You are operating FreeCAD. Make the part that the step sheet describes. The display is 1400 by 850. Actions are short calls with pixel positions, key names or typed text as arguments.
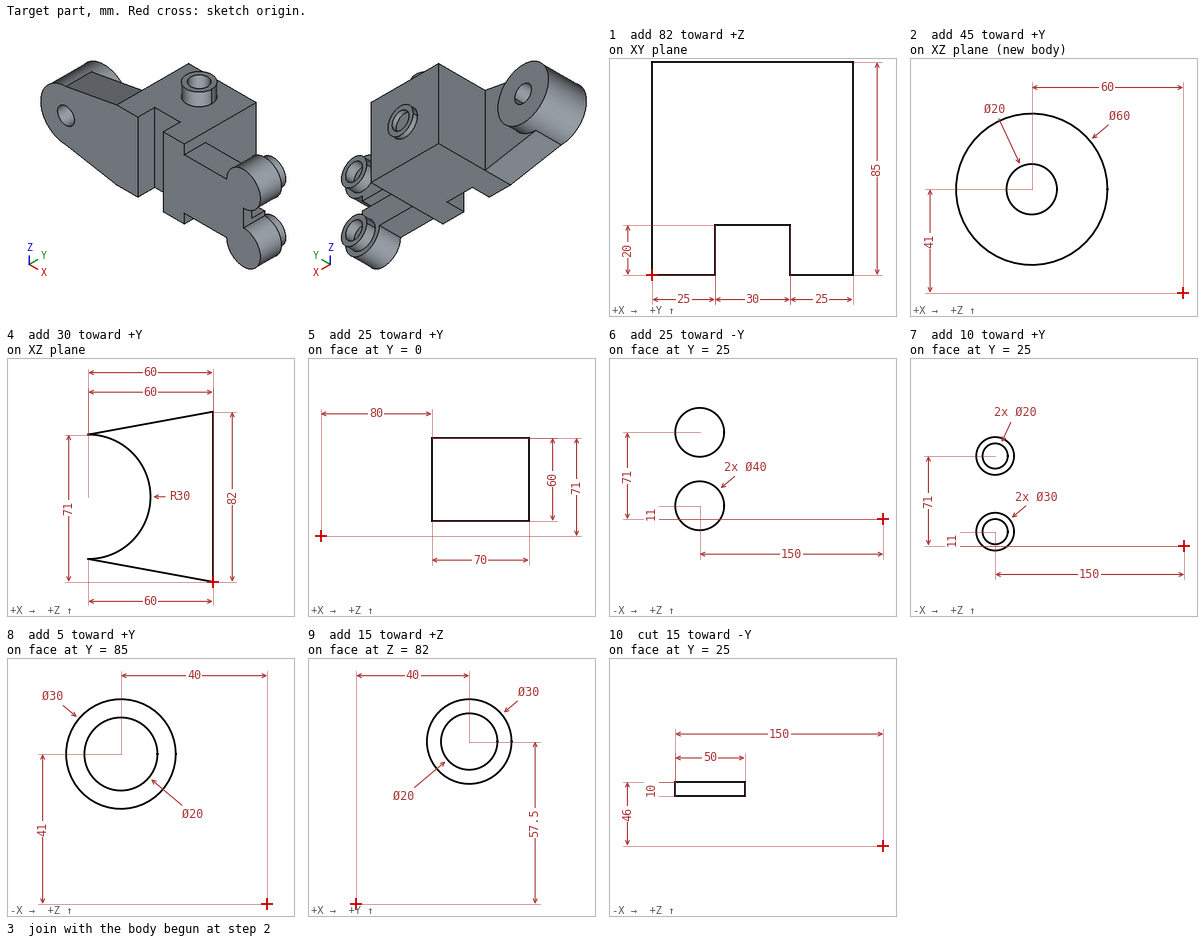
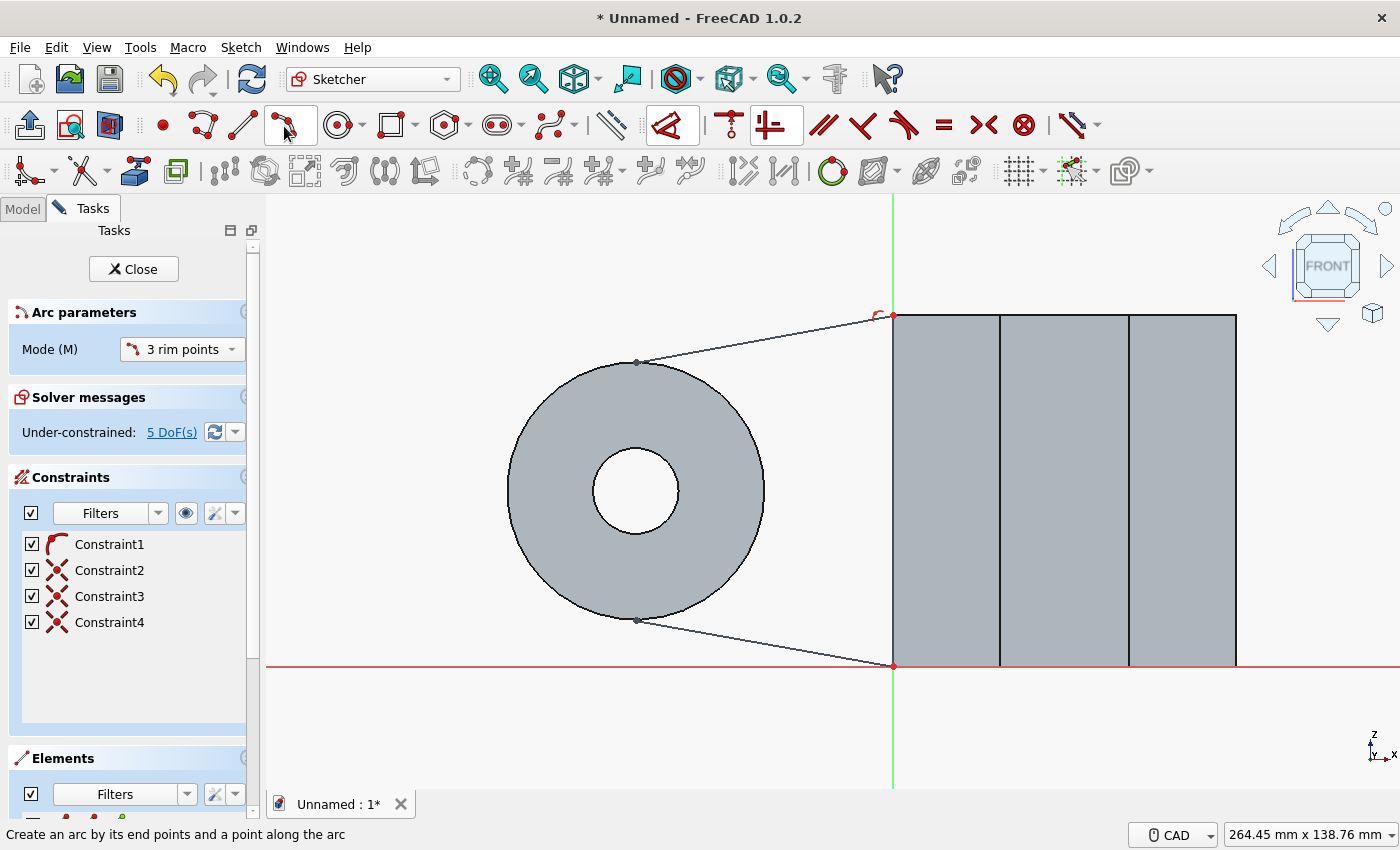
click(636, 621)
click(636, 363)
click(764, 491)
key(Escape)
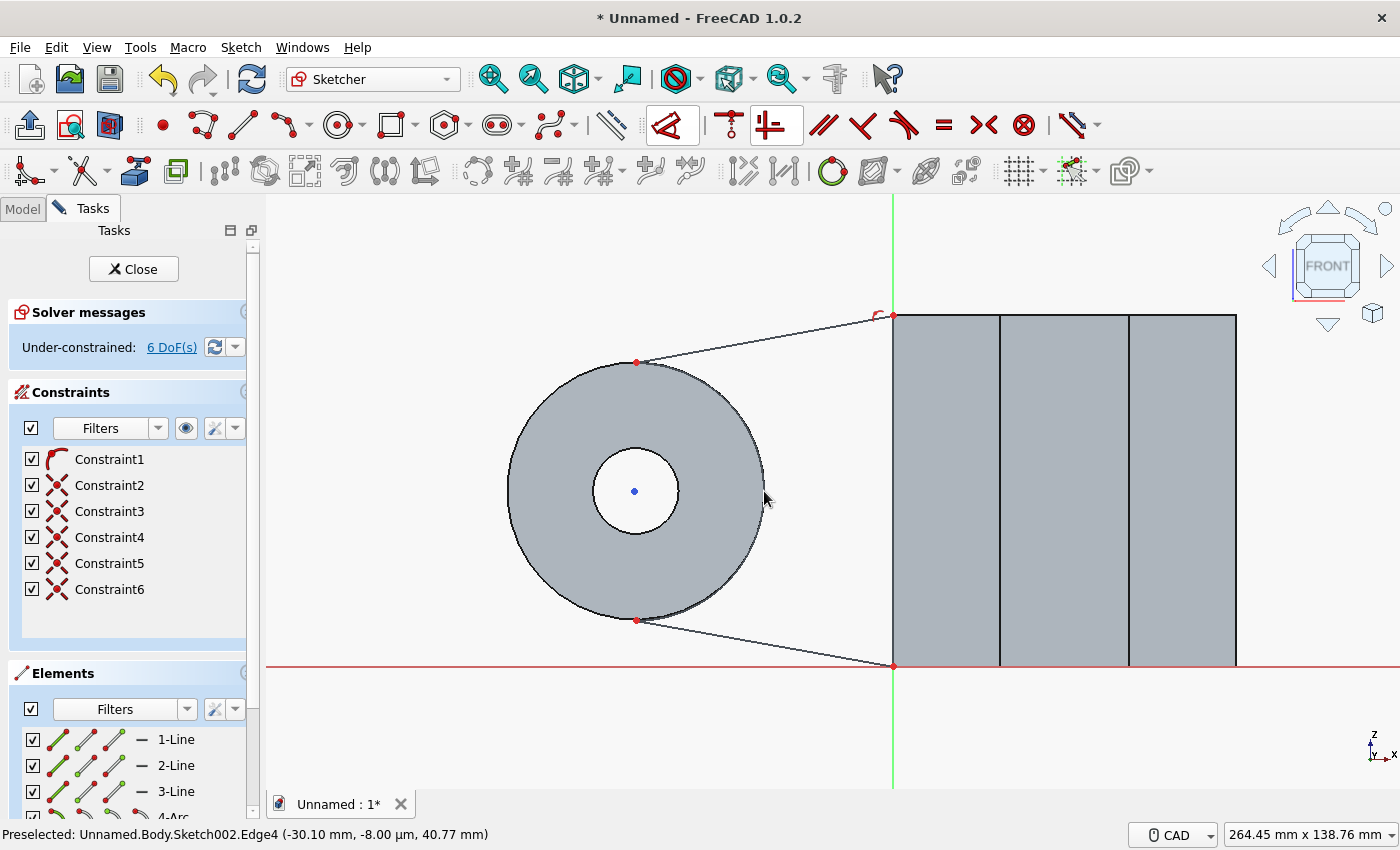
click(740, 568)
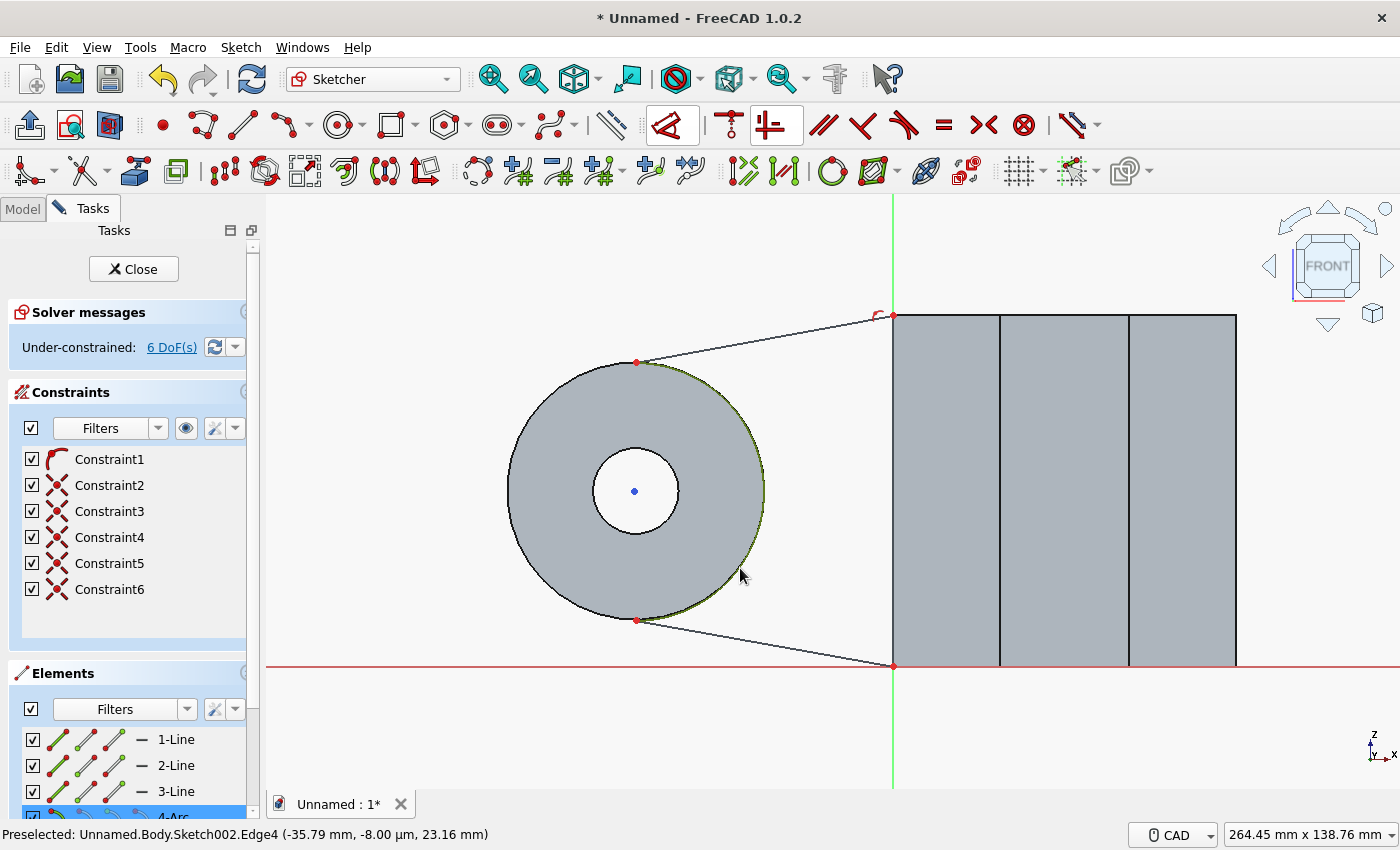
key(k)
key(r)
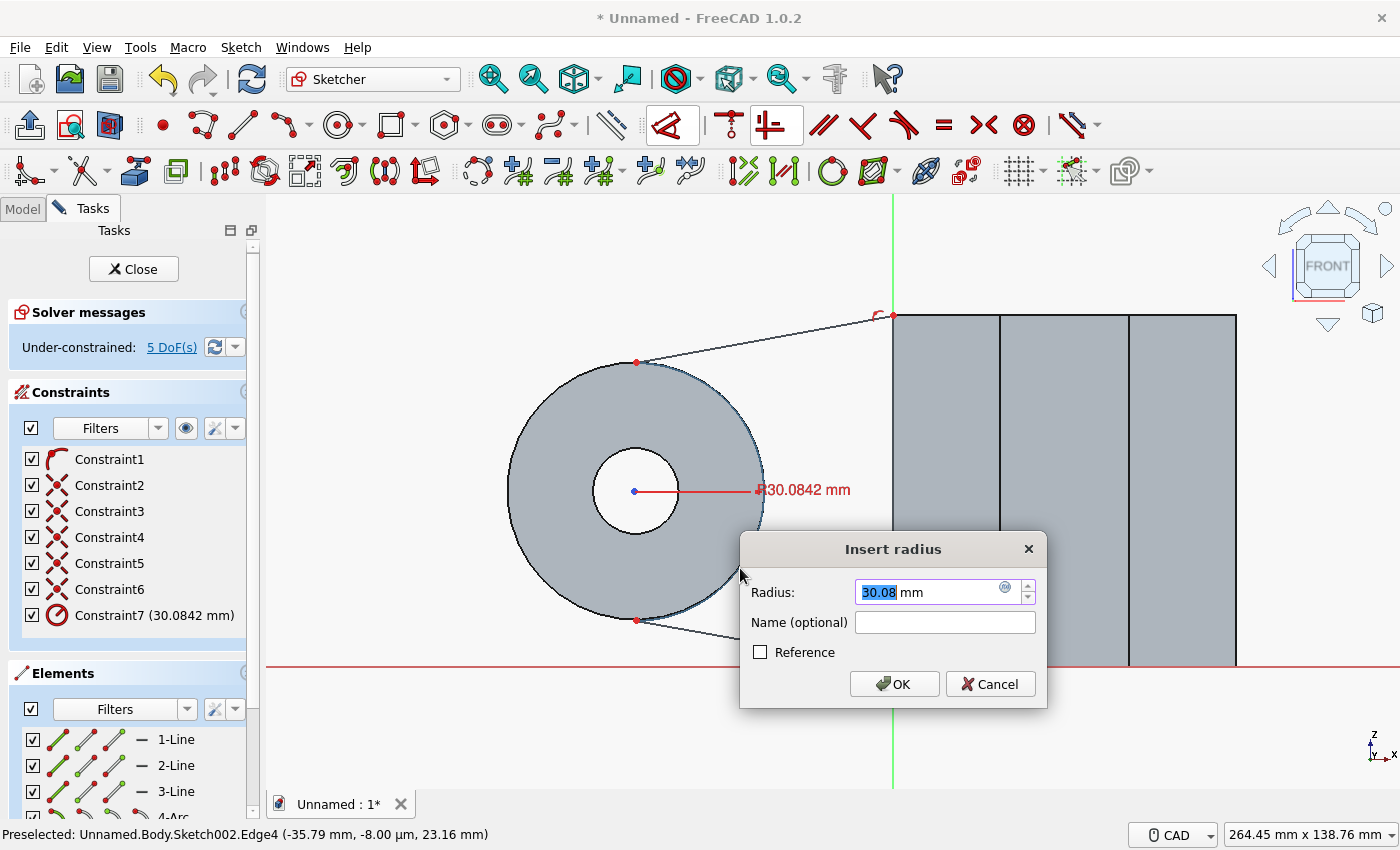
text(30)
key(Return)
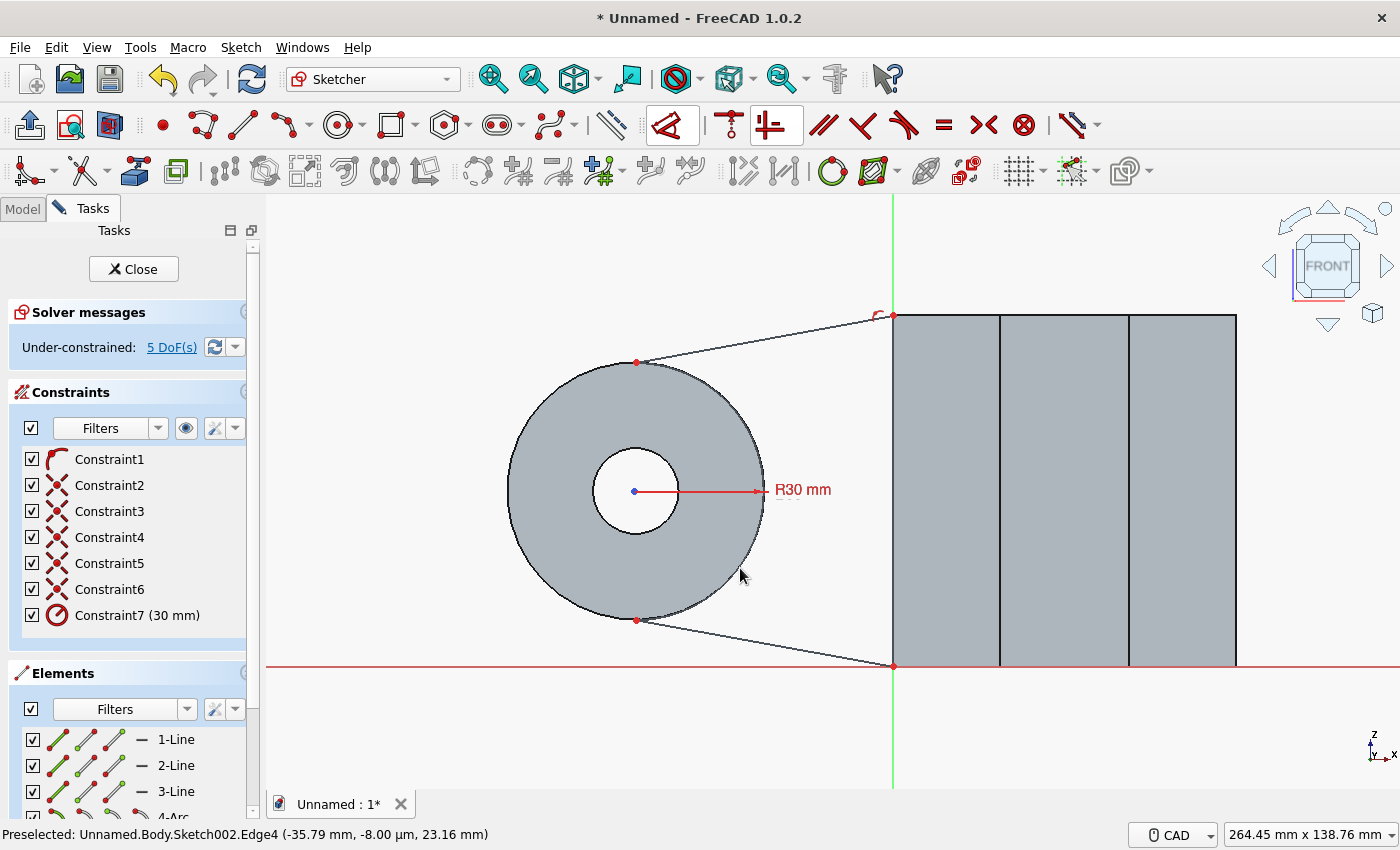
click(893, 421)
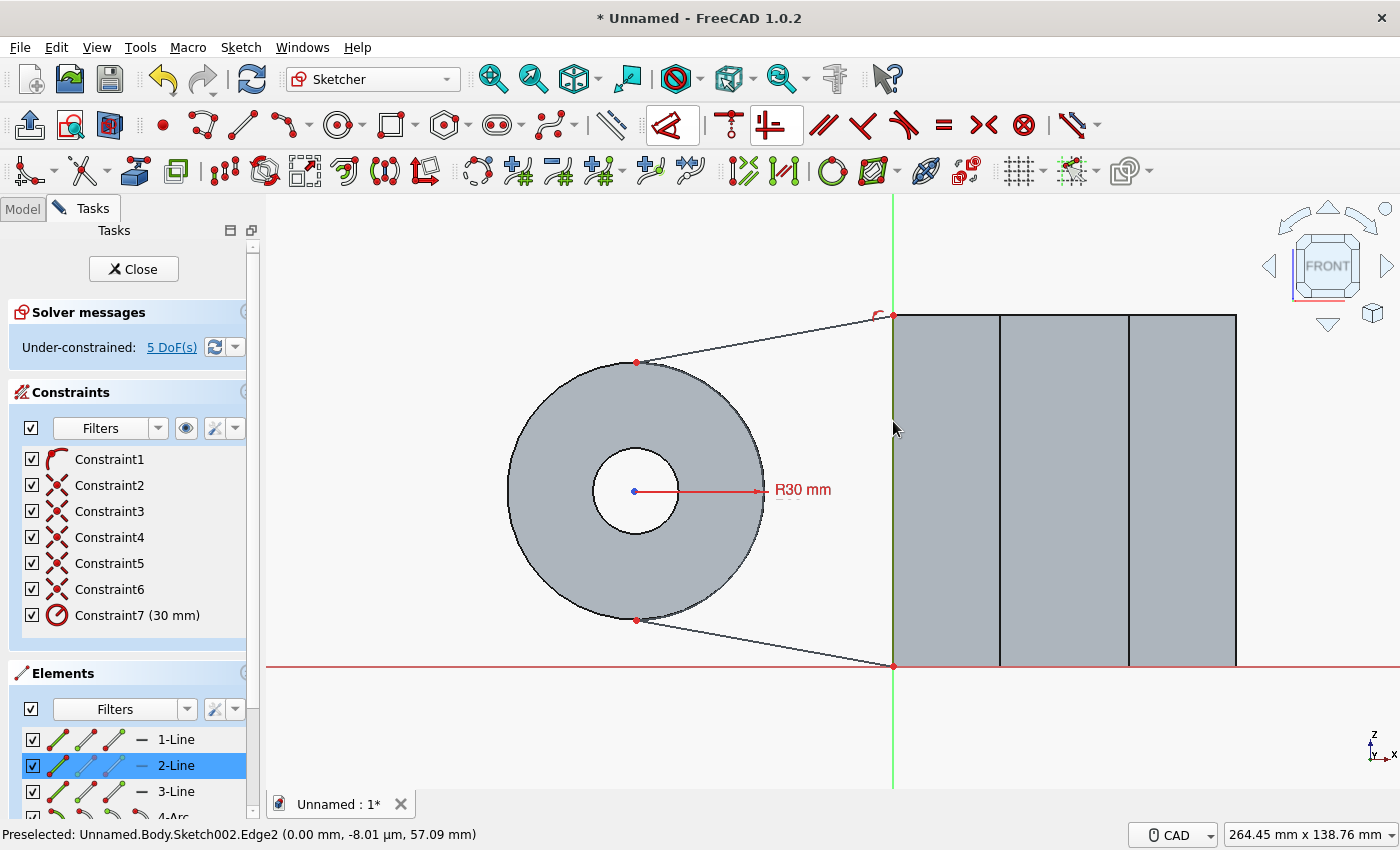
click(694, 126)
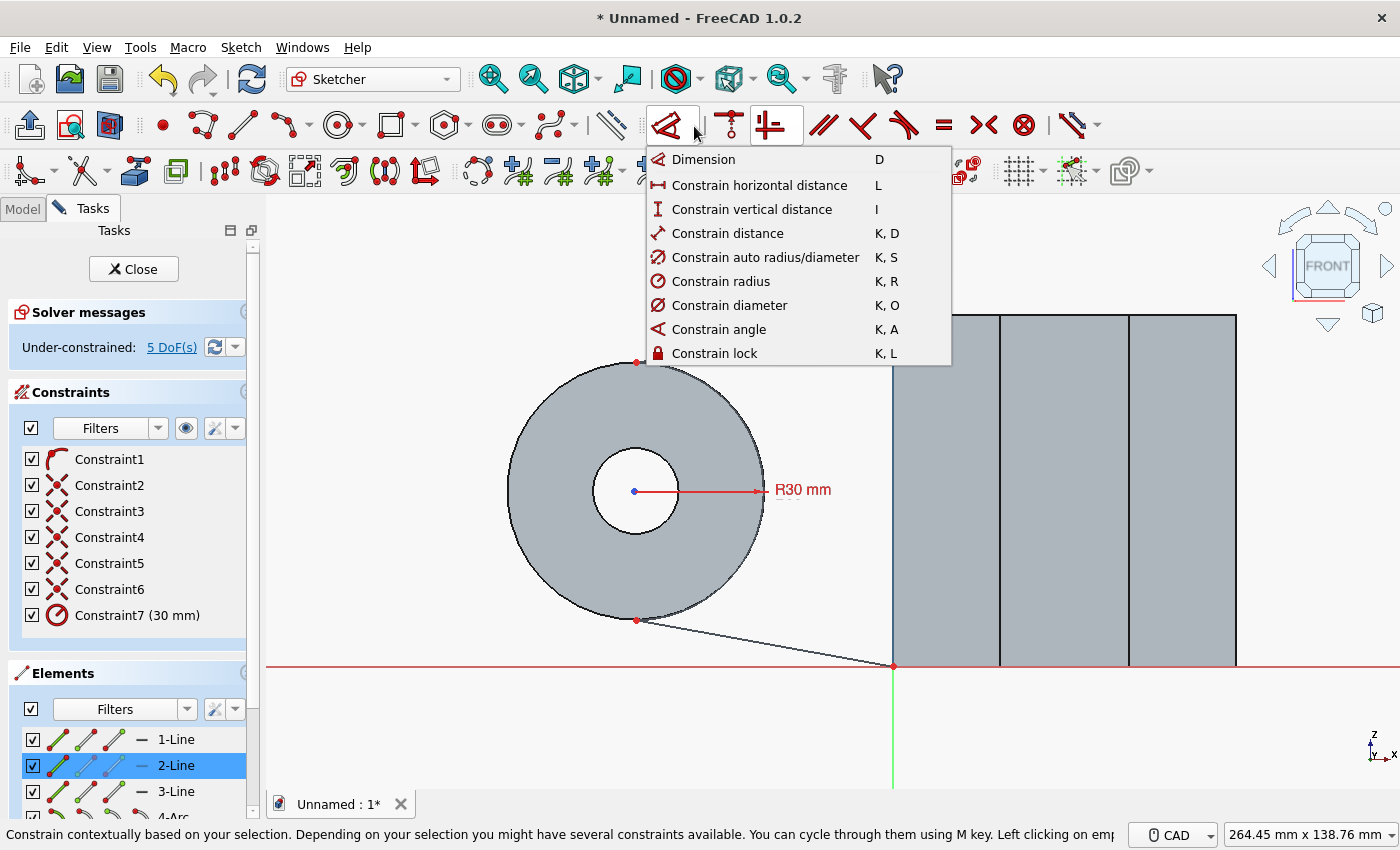
click(799, 209)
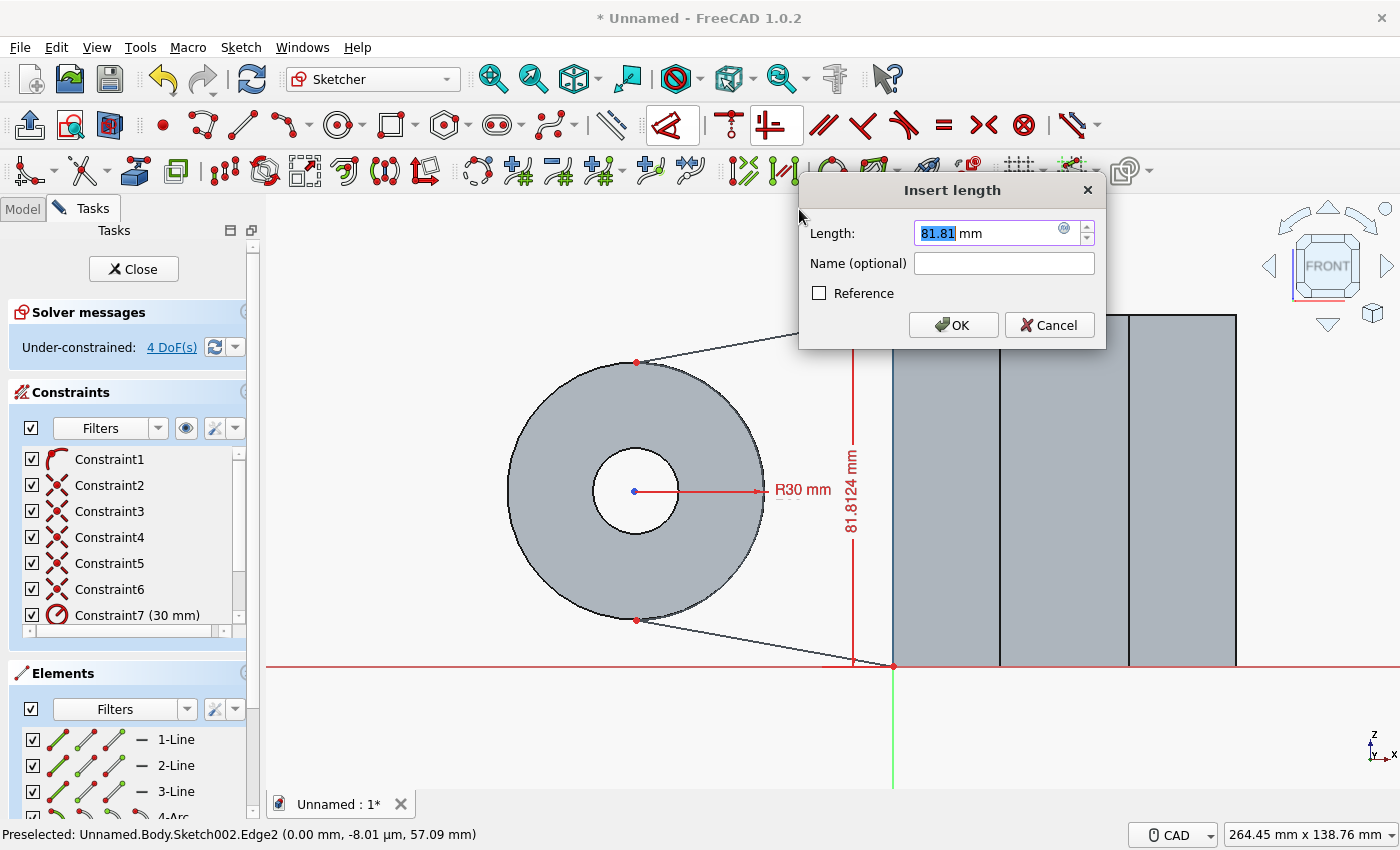
text(82)
key(Return)